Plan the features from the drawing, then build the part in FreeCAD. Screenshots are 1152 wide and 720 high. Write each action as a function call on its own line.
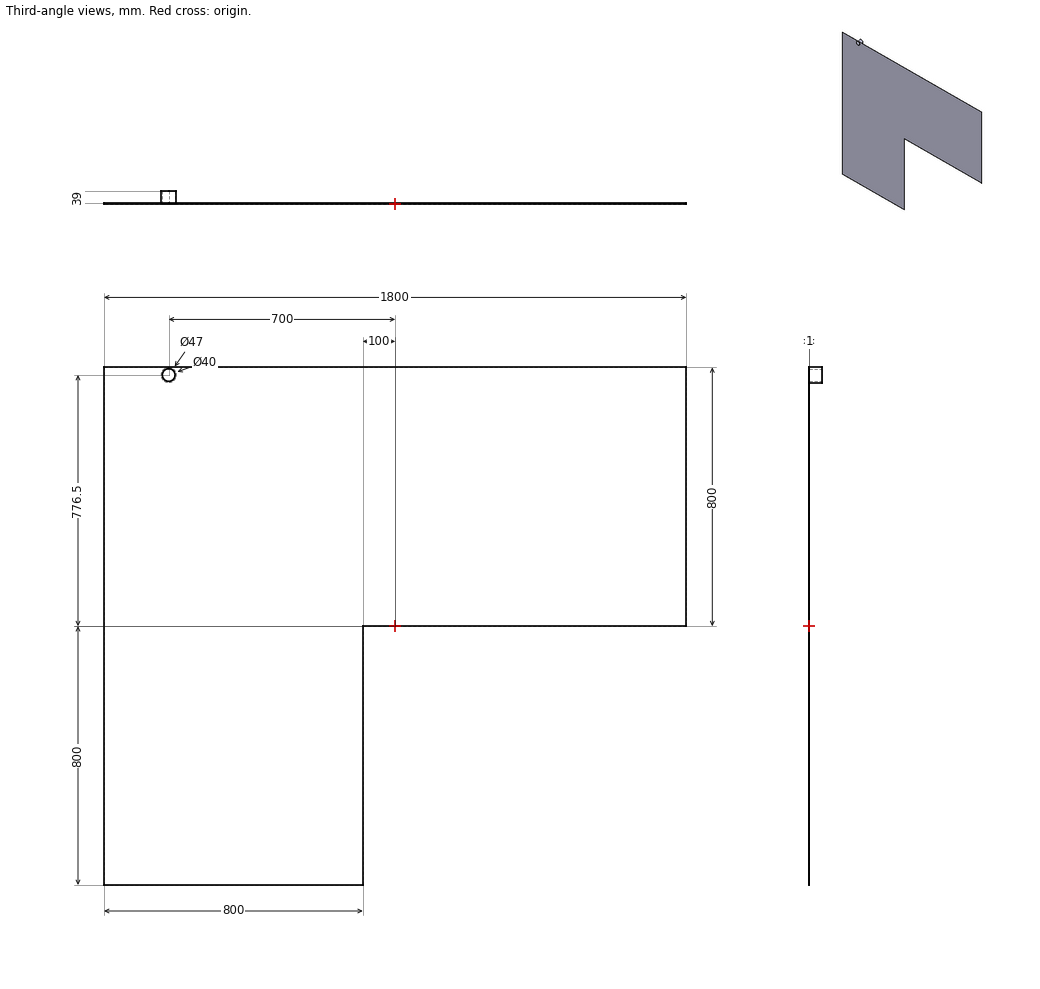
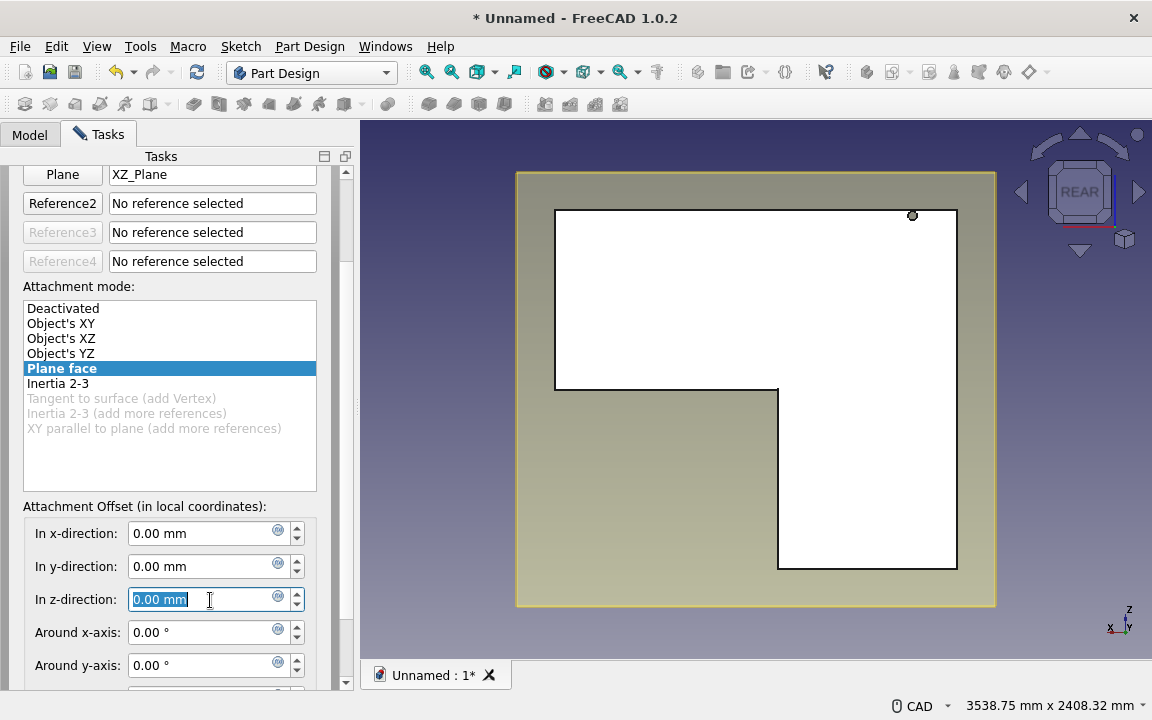
text(-40)
key(Tab)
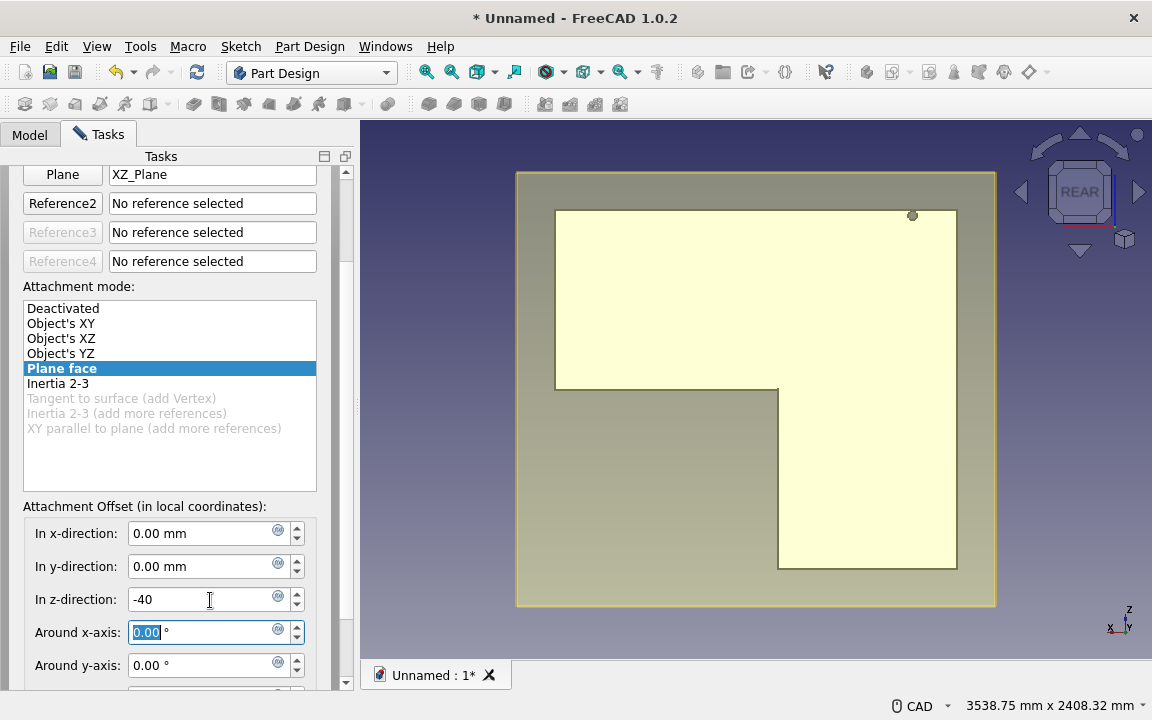
scroll(346, 428, up, 3)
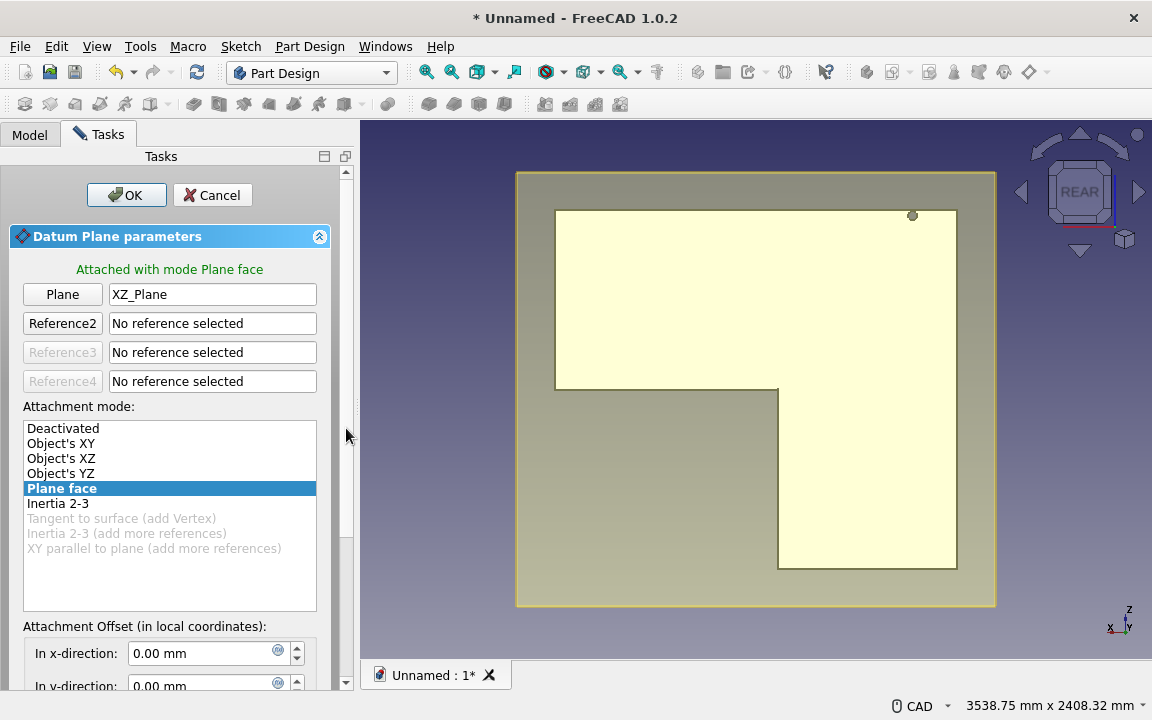
click(127, 195)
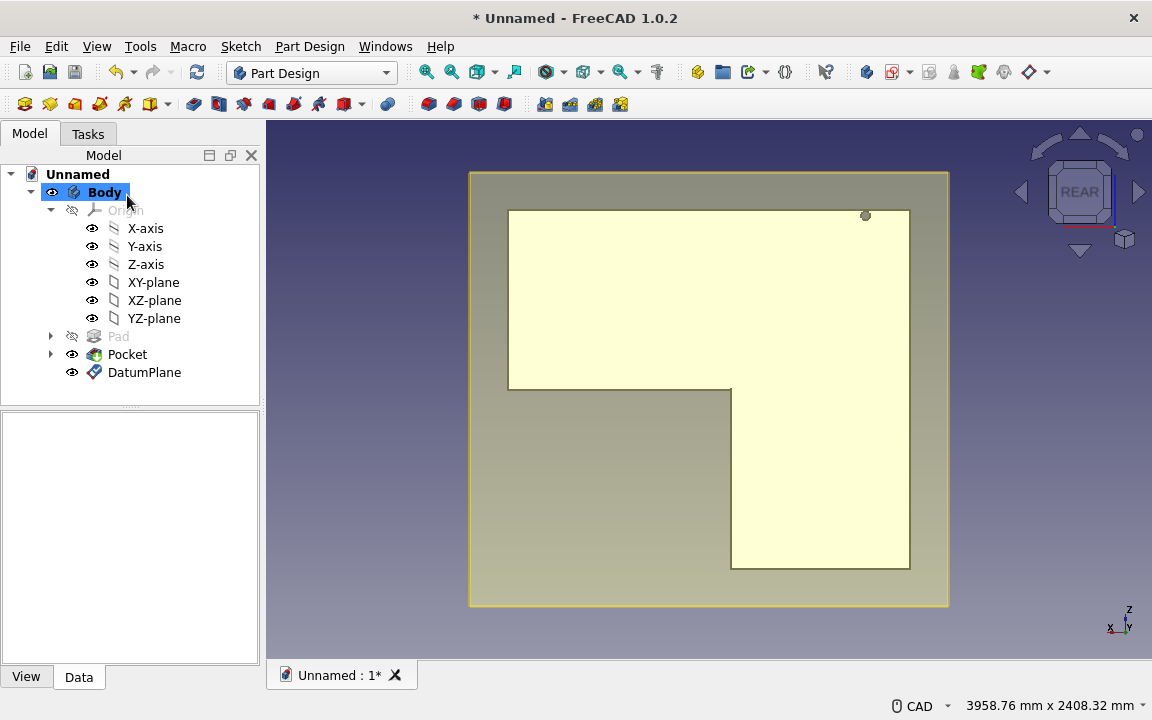
click(117, 372)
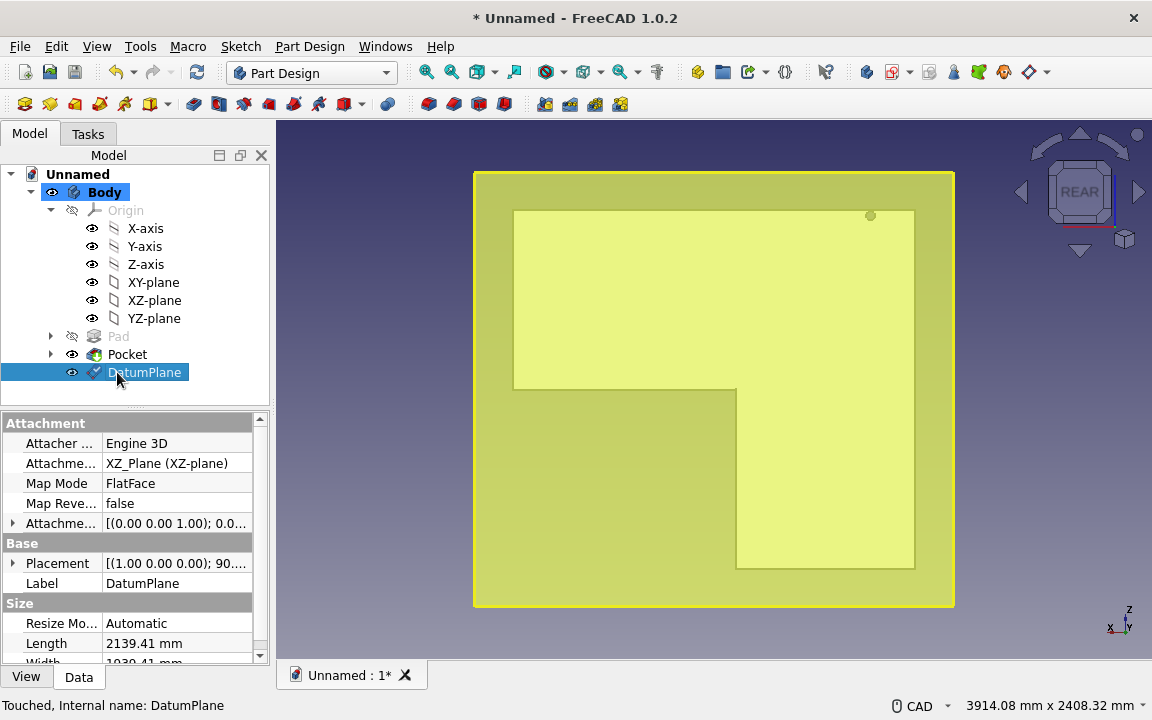
click(892, 72)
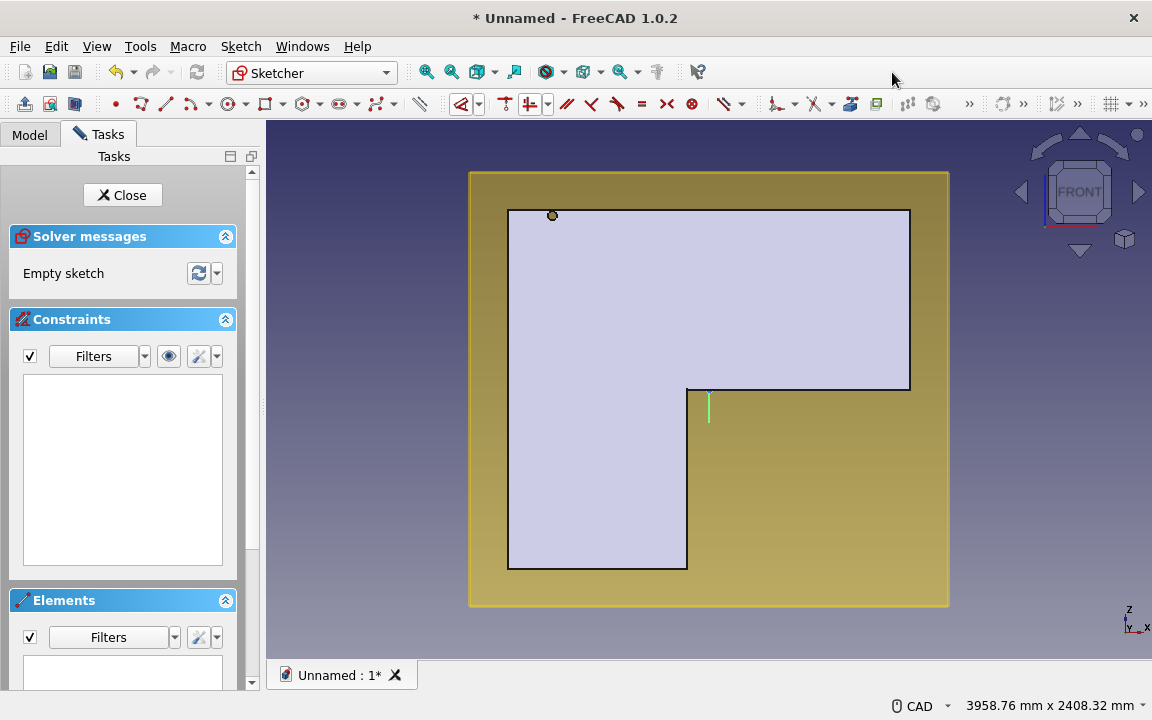
click(75, 104)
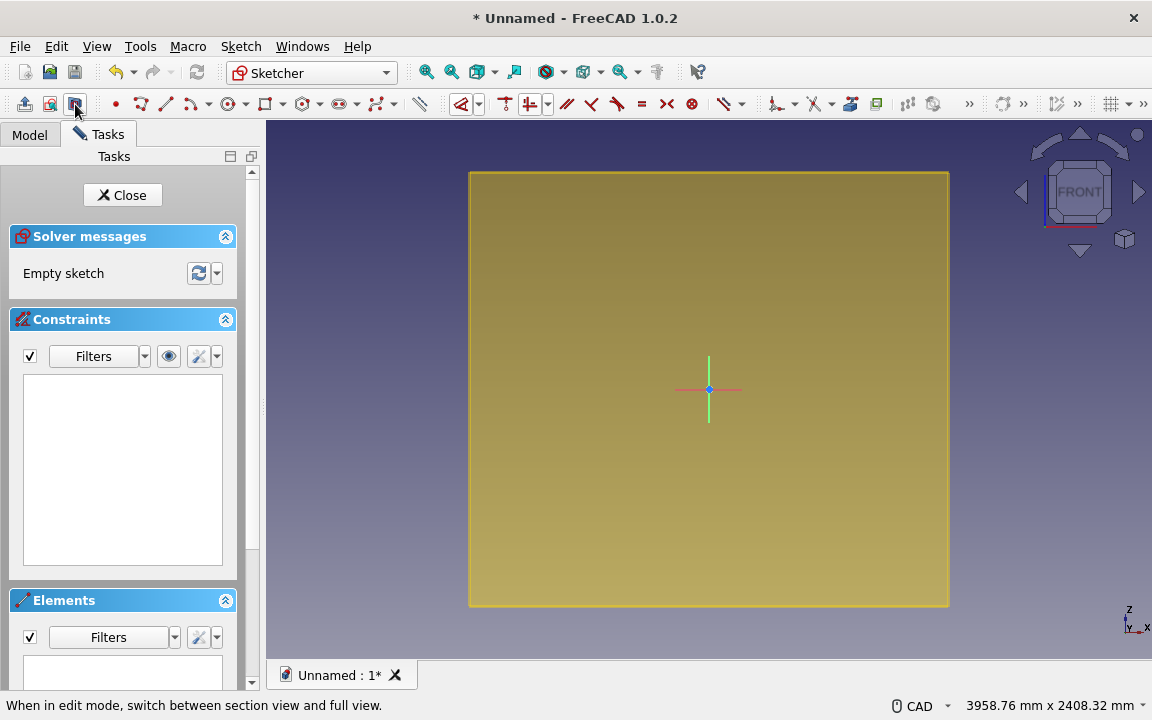
scroll(548, 207, up, 15)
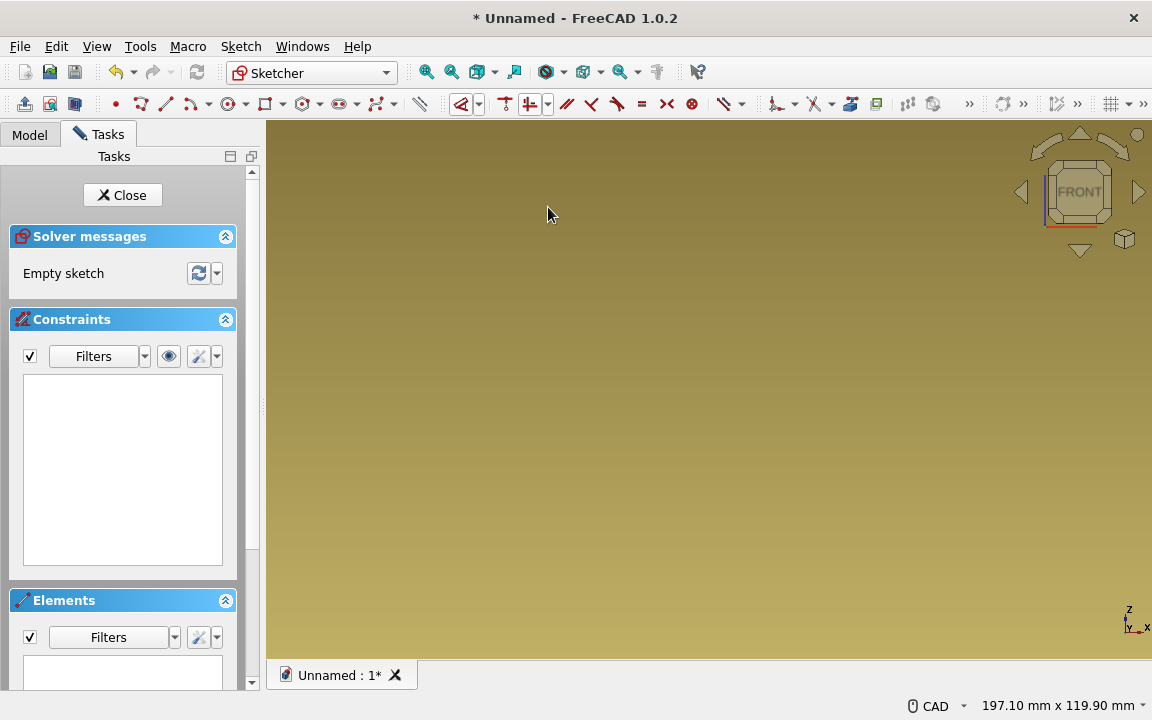
scroll(606, 357, up, 2)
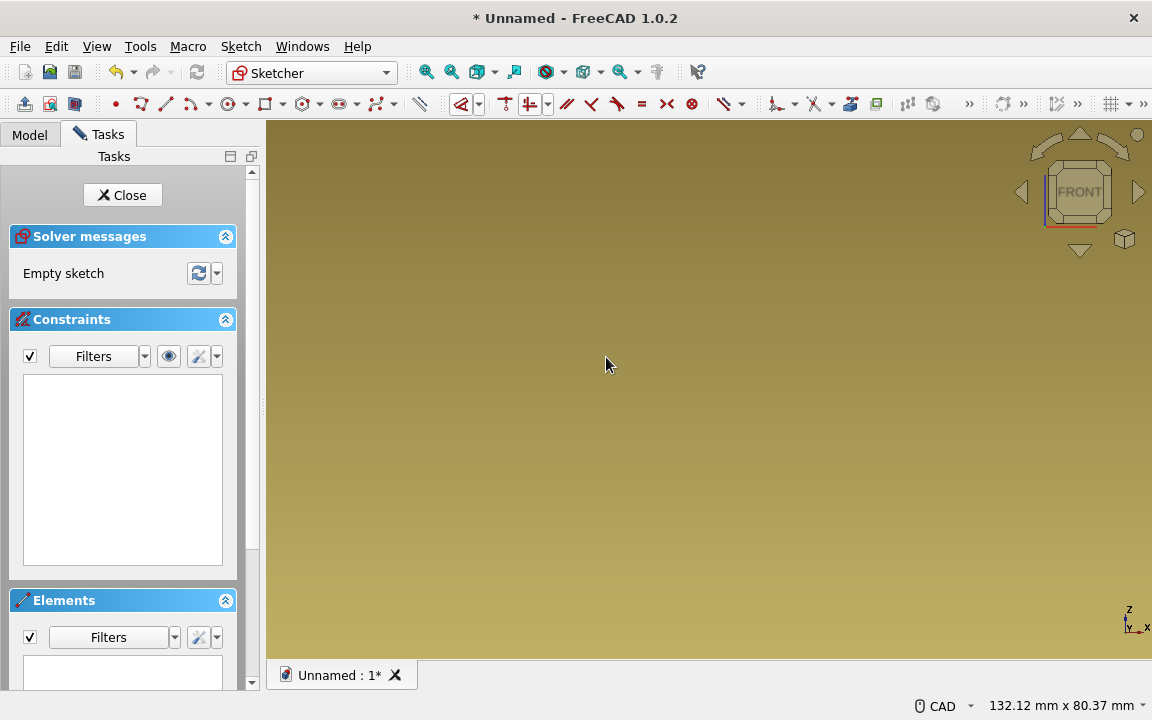
click(228, 104)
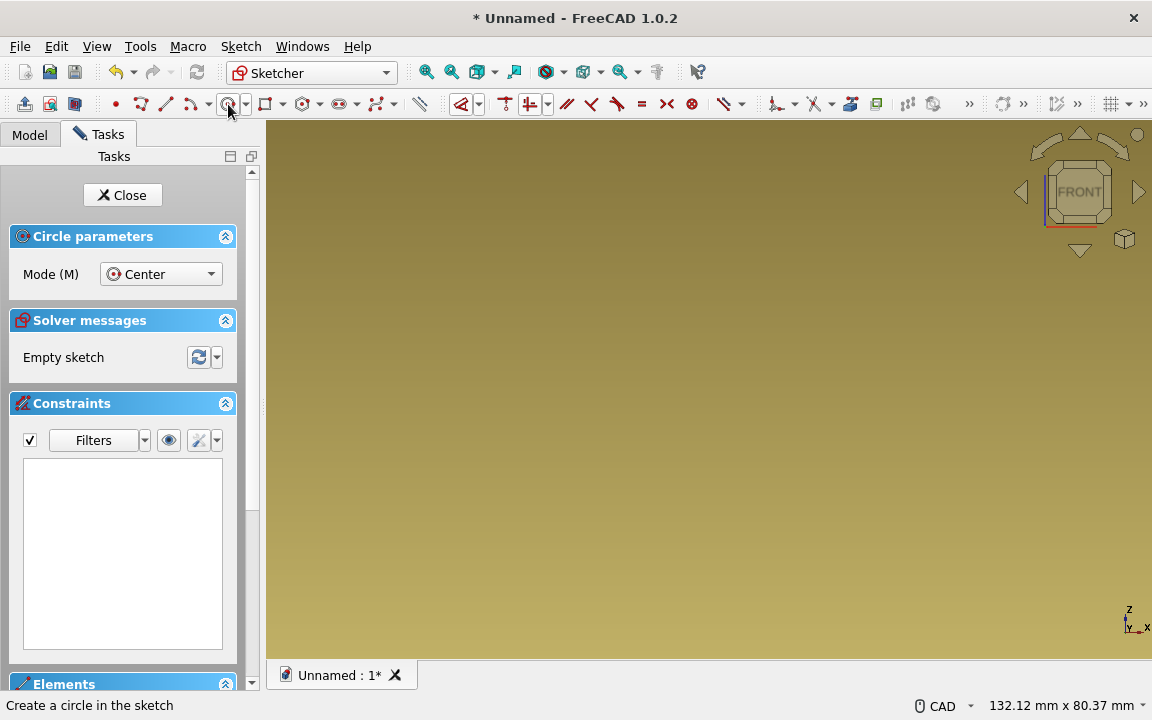
click(640, 389)
click(752, 278)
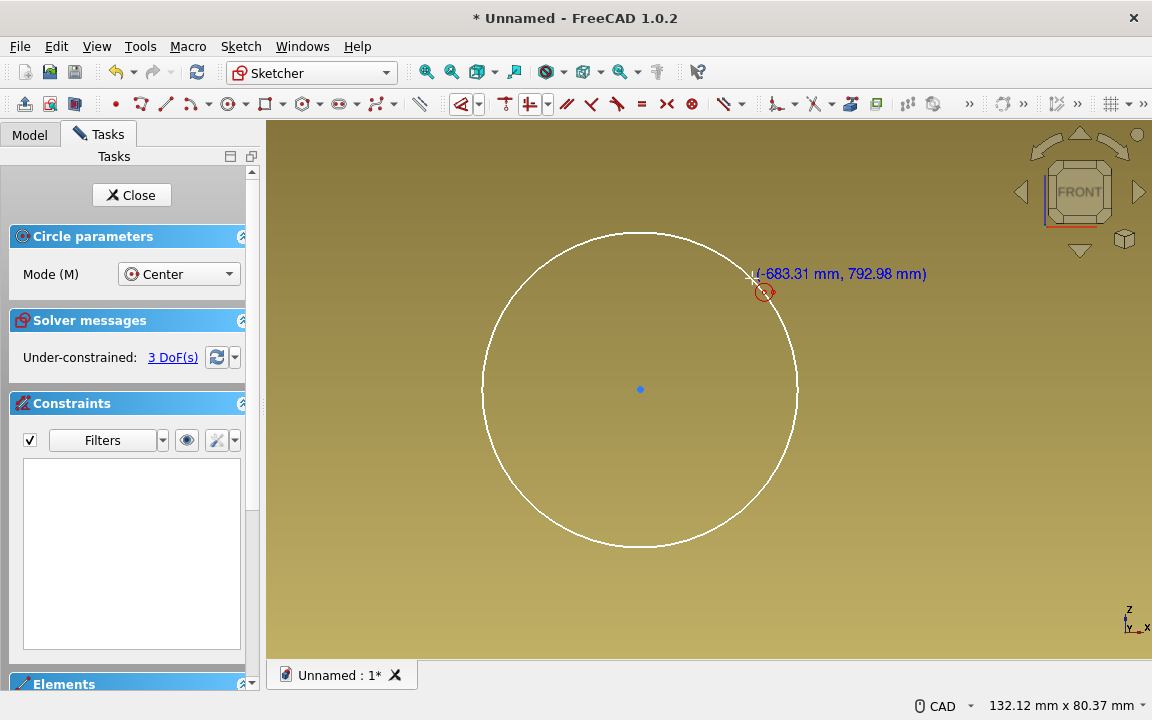
click(640, 390)
click(735, 295)
key(Escape)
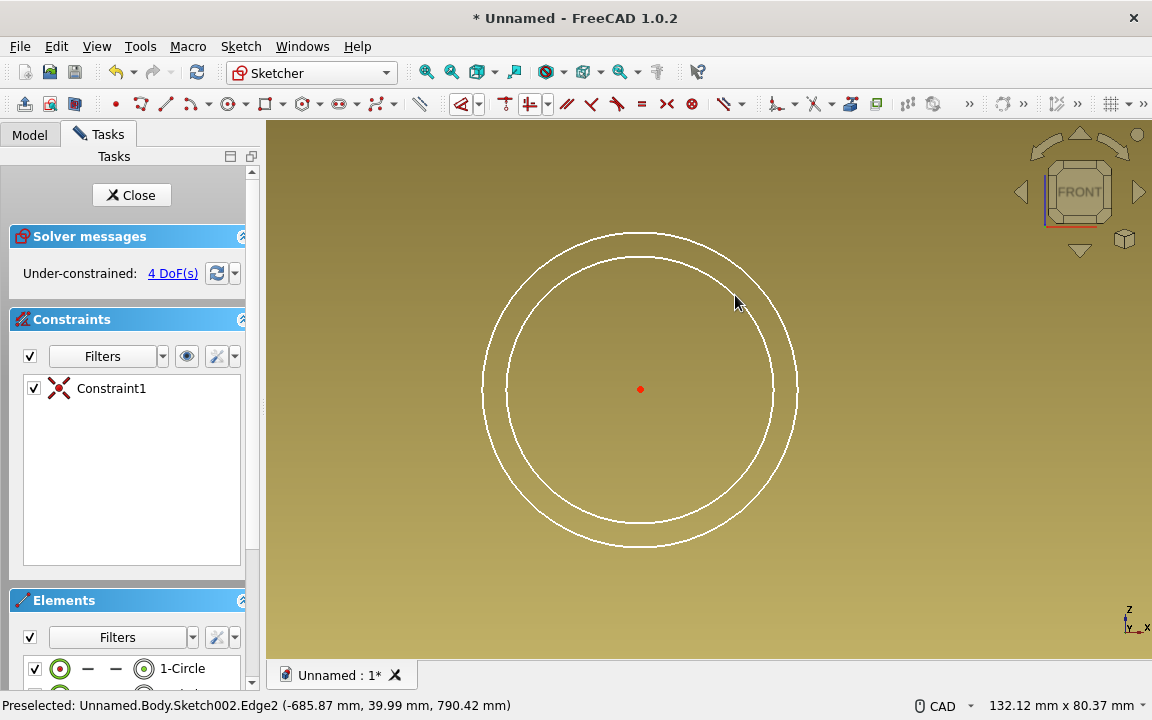
click(751, 278)